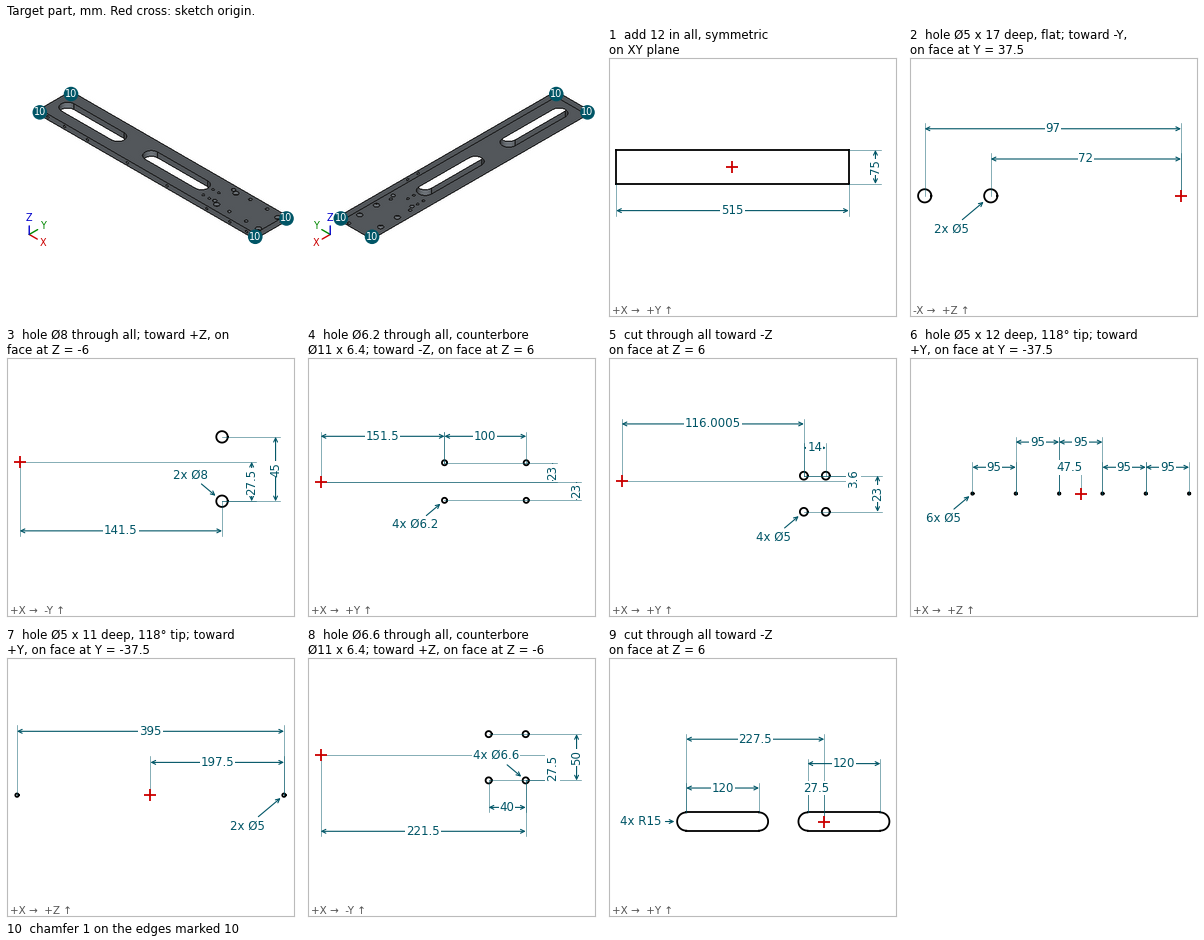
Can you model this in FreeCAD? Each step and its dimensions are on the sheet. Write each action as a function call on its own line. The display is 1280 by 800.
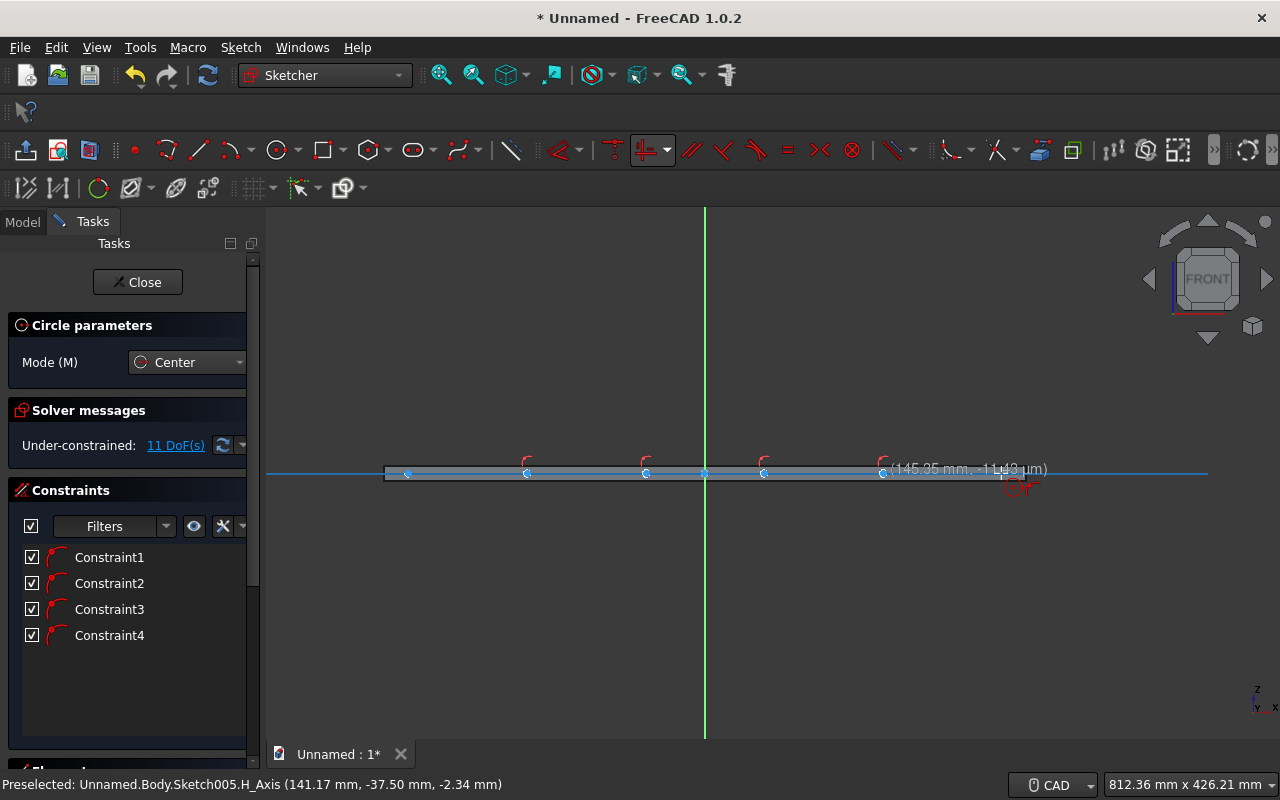
click(1001, 473)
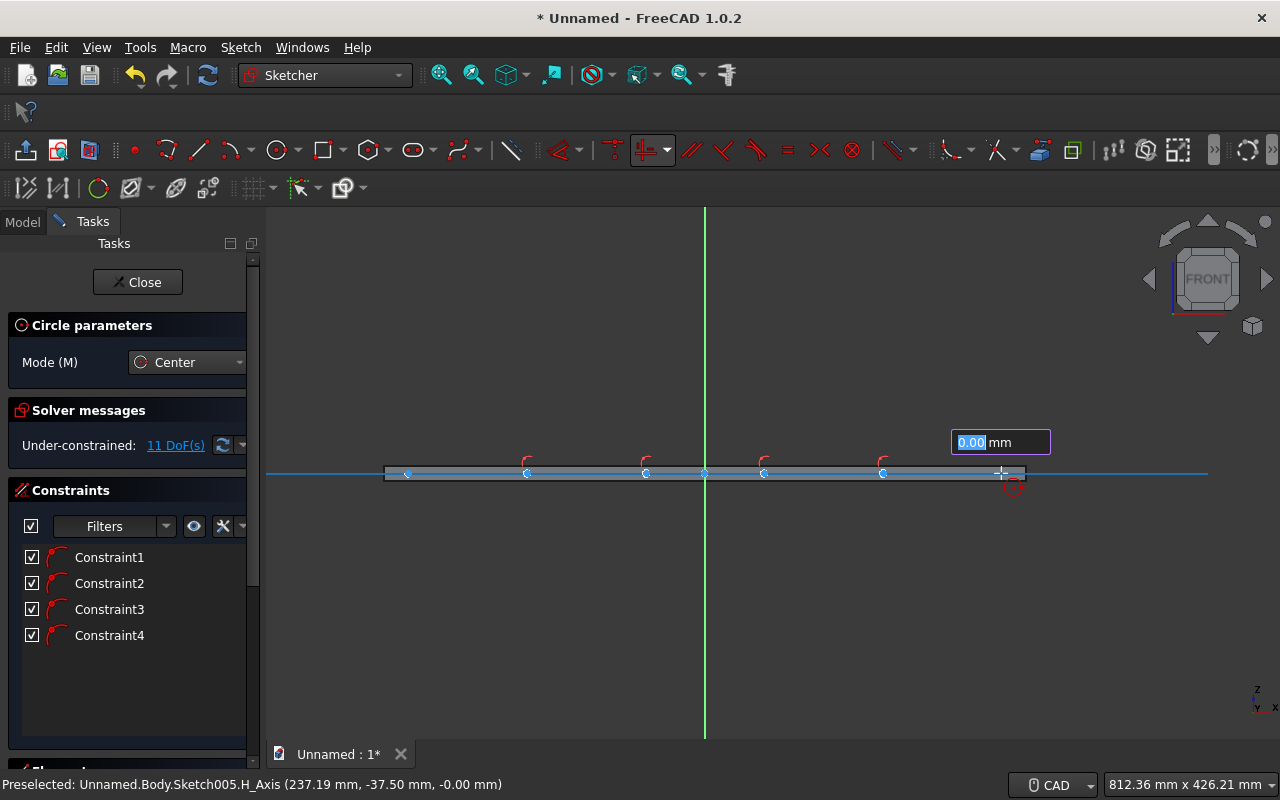
scroll(1000, 476, up, 9)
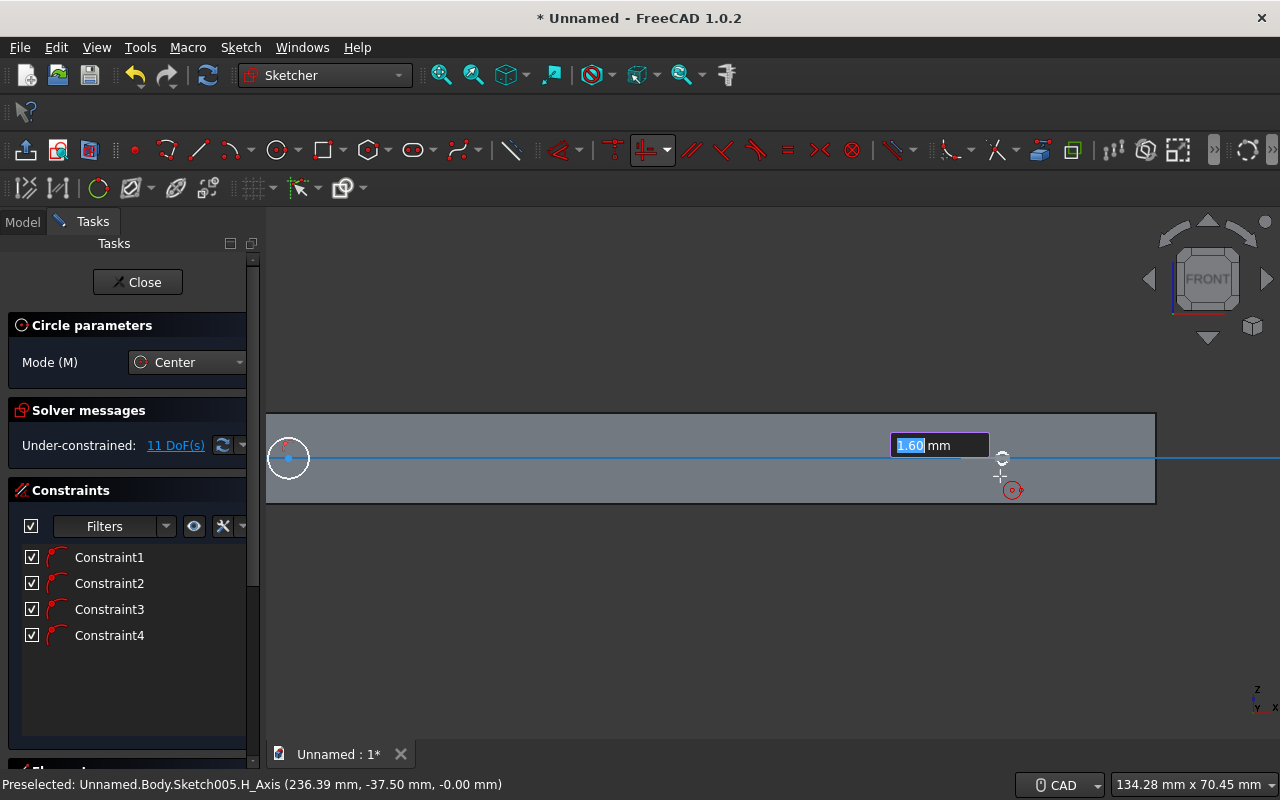
click(998, 476)
key(Escape)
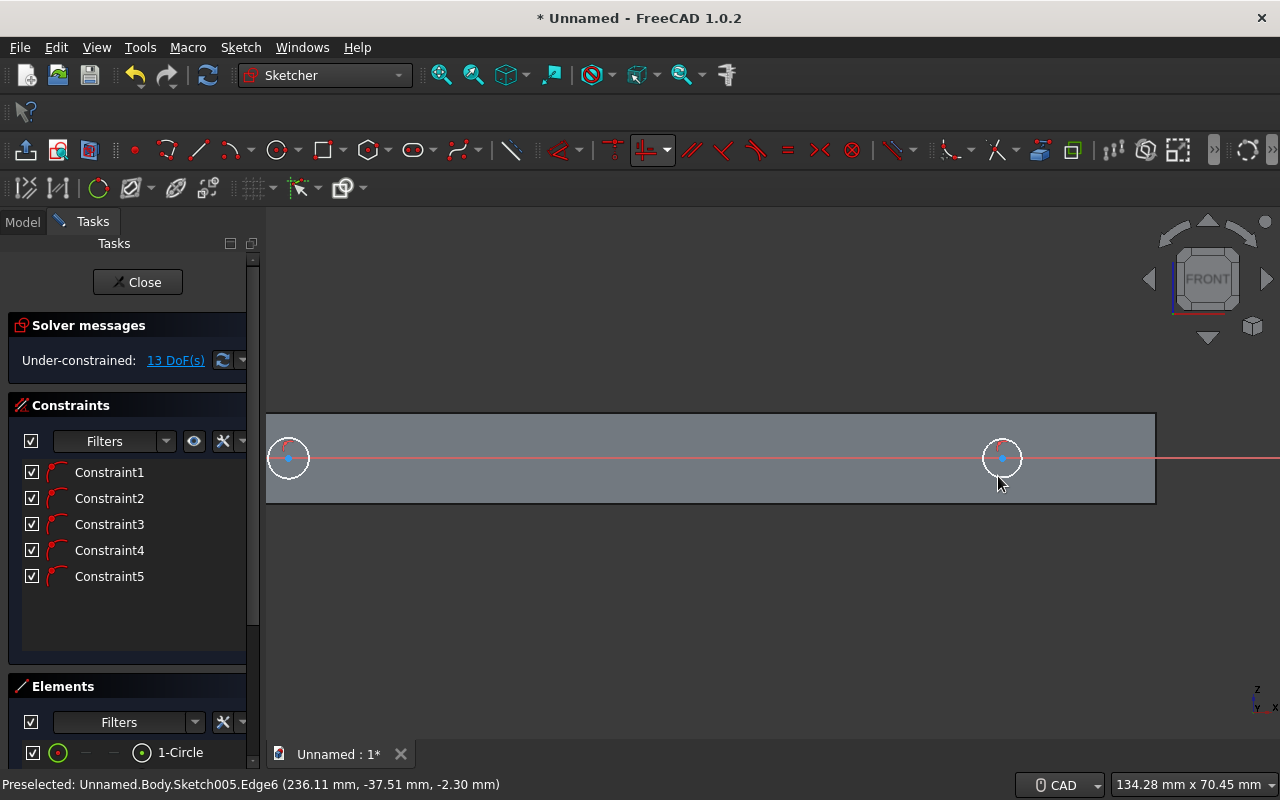
scroll(1000, 476, down, 9)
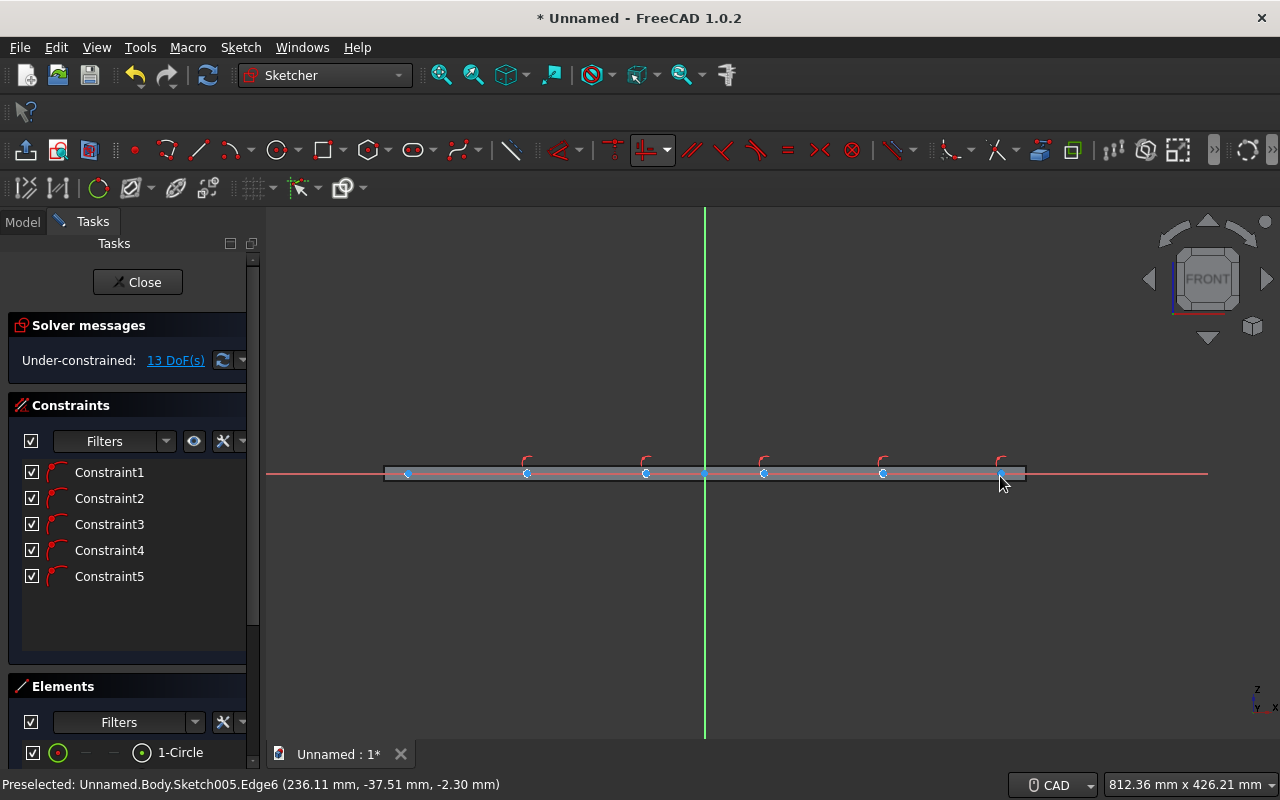
scroll(406, 476, up, 9)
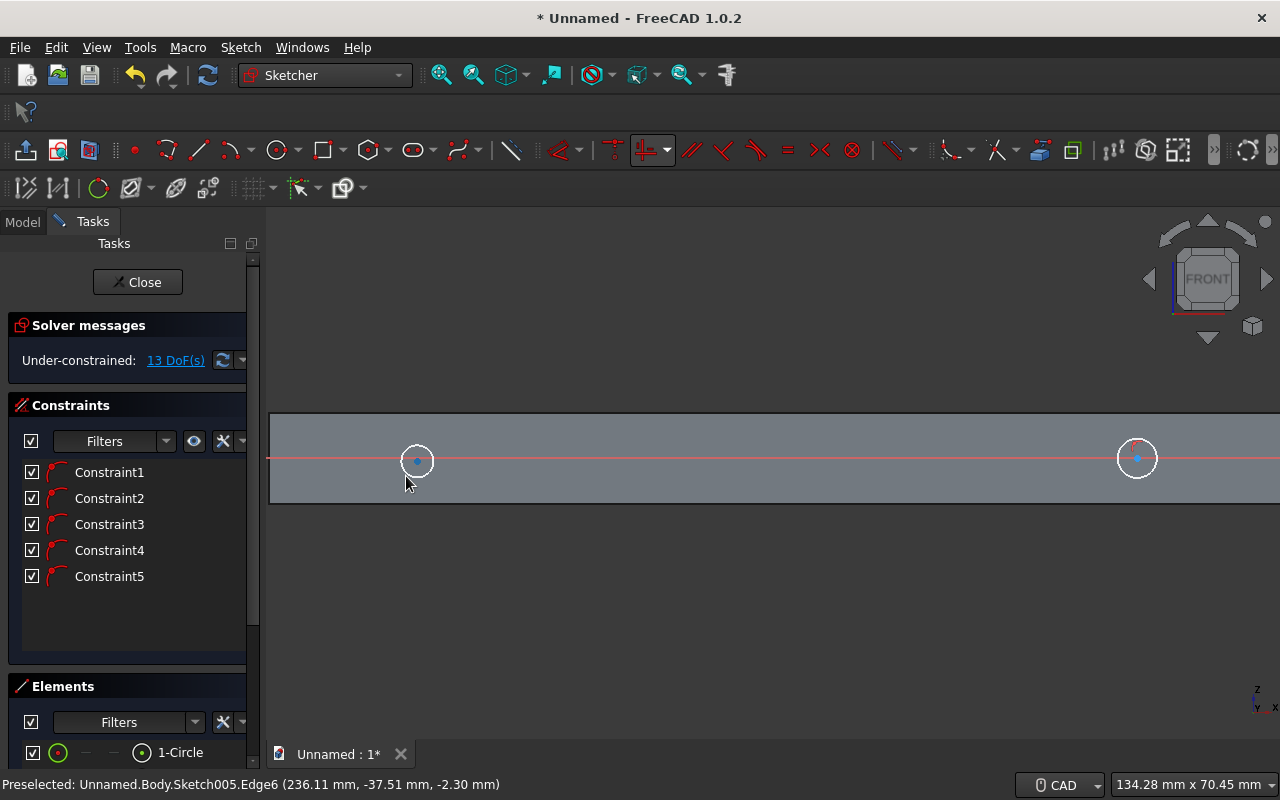
click(406, 473)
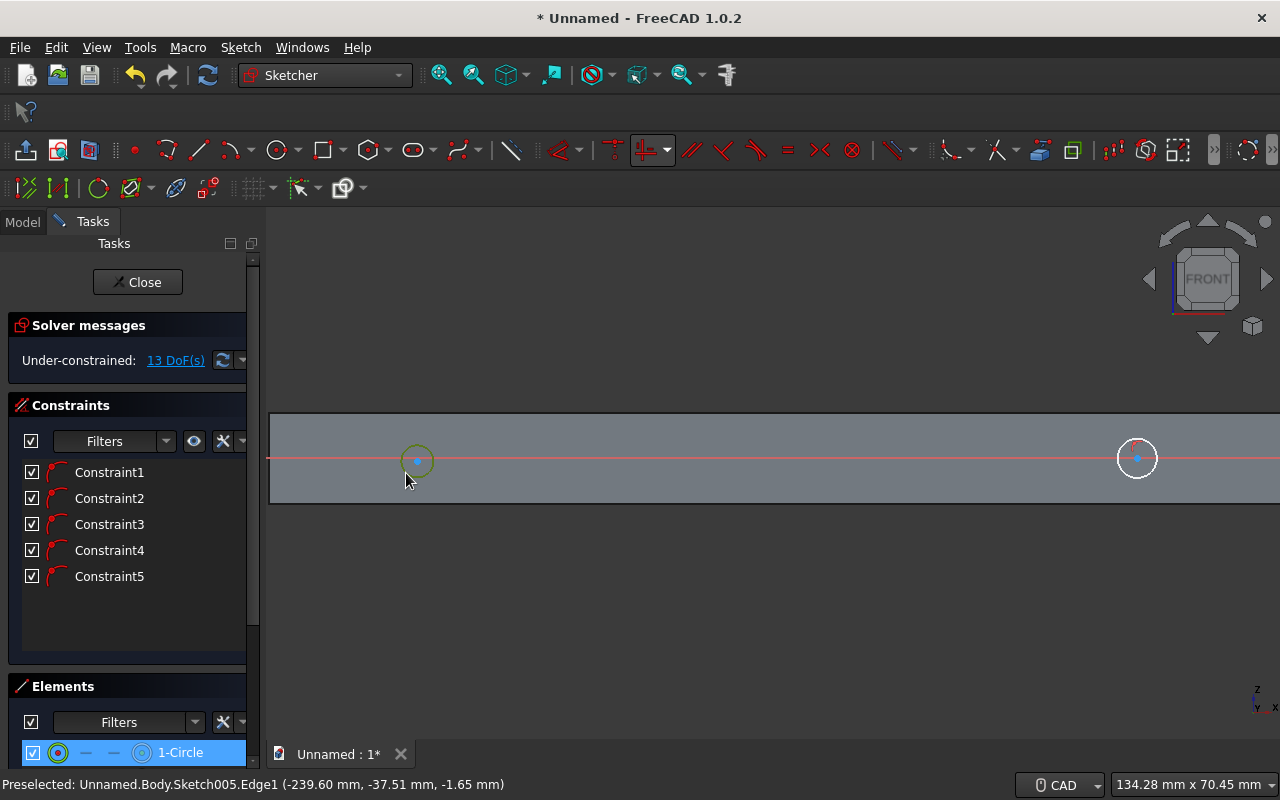
scroll(406, 476, down, 9)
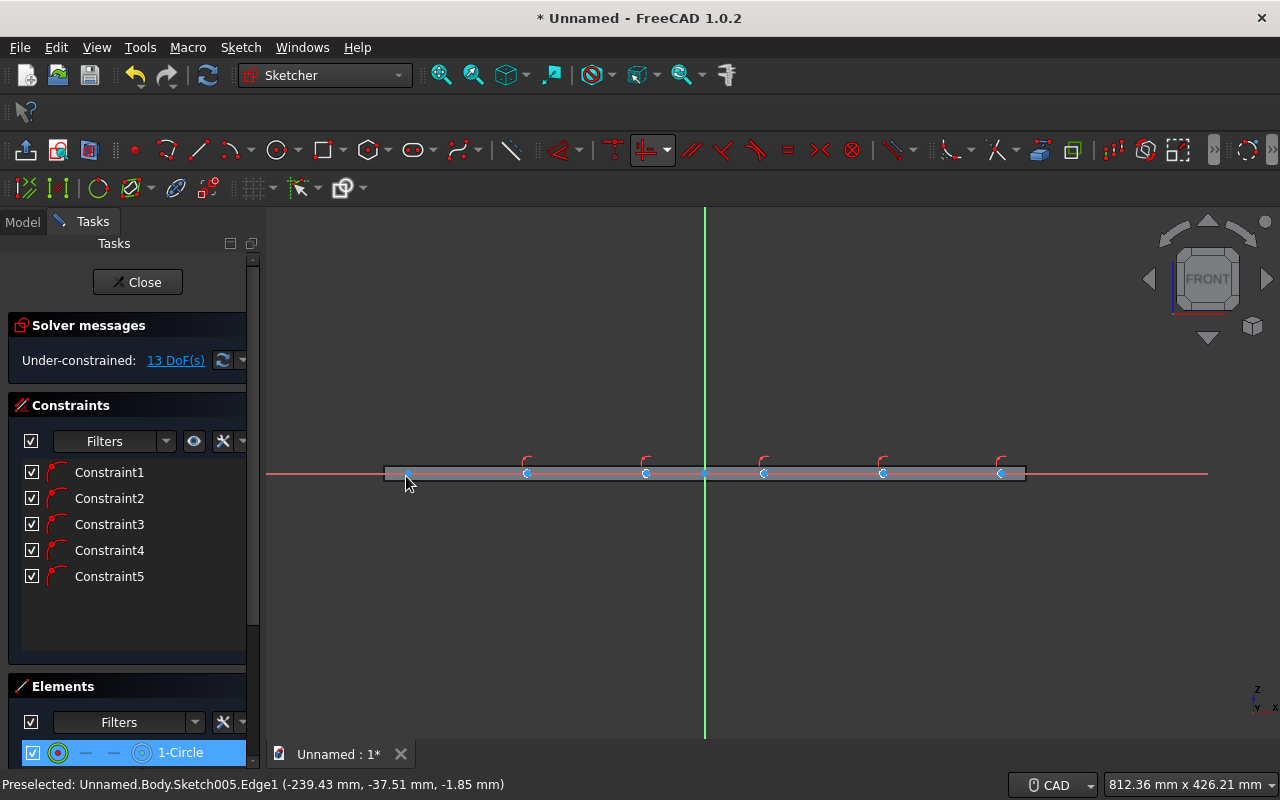
scroll(529, 471, up, 9)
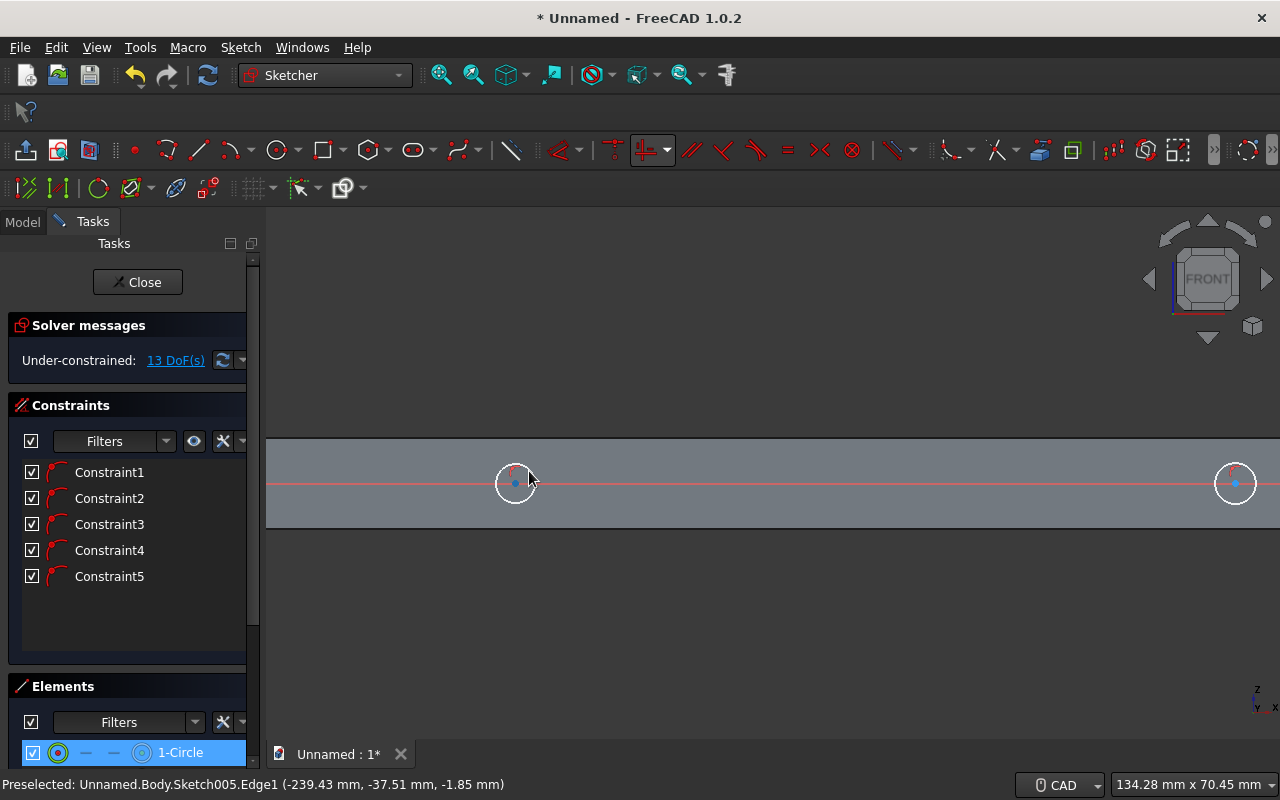
click(529, 470)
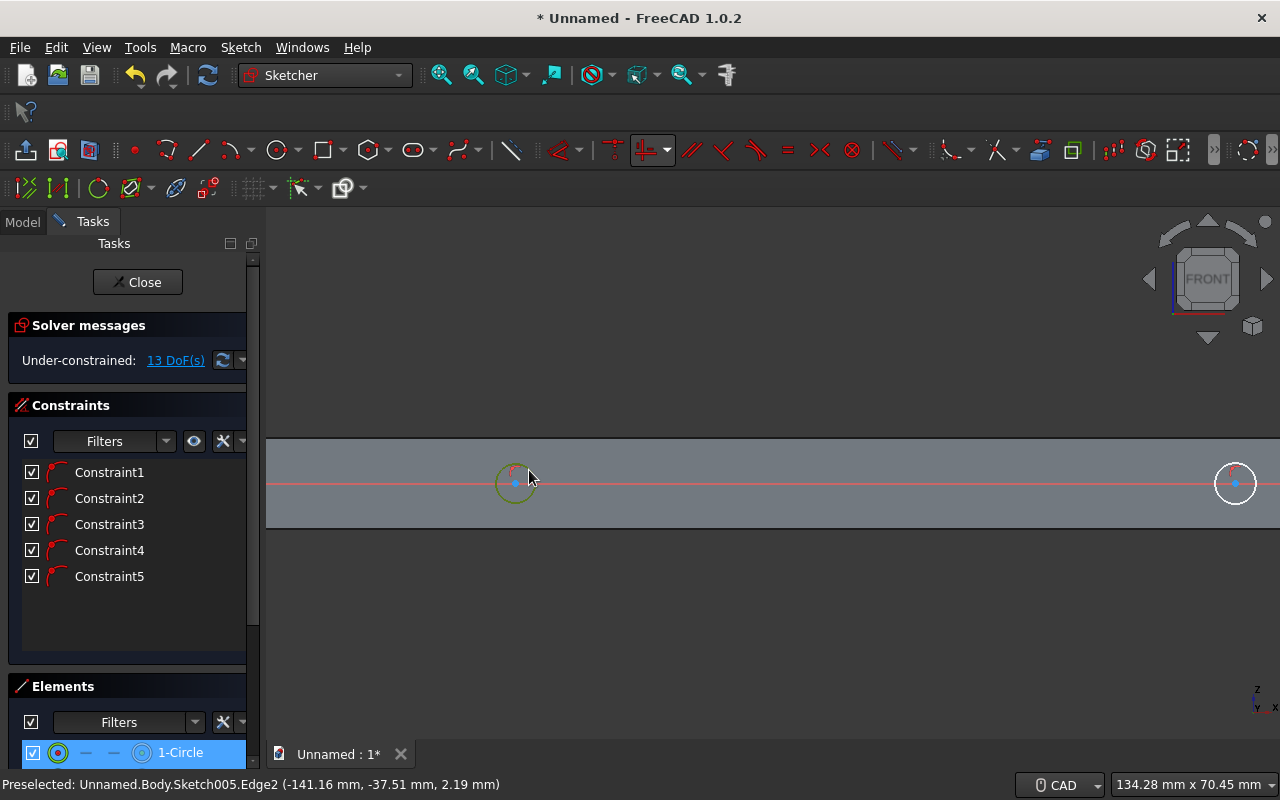
scroll(529, 471, down, 9)